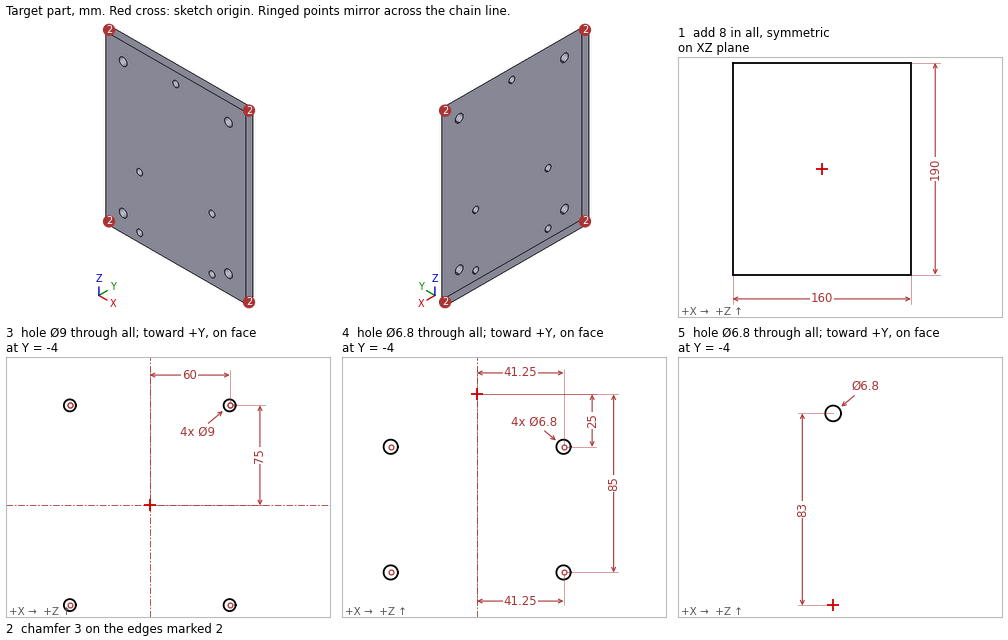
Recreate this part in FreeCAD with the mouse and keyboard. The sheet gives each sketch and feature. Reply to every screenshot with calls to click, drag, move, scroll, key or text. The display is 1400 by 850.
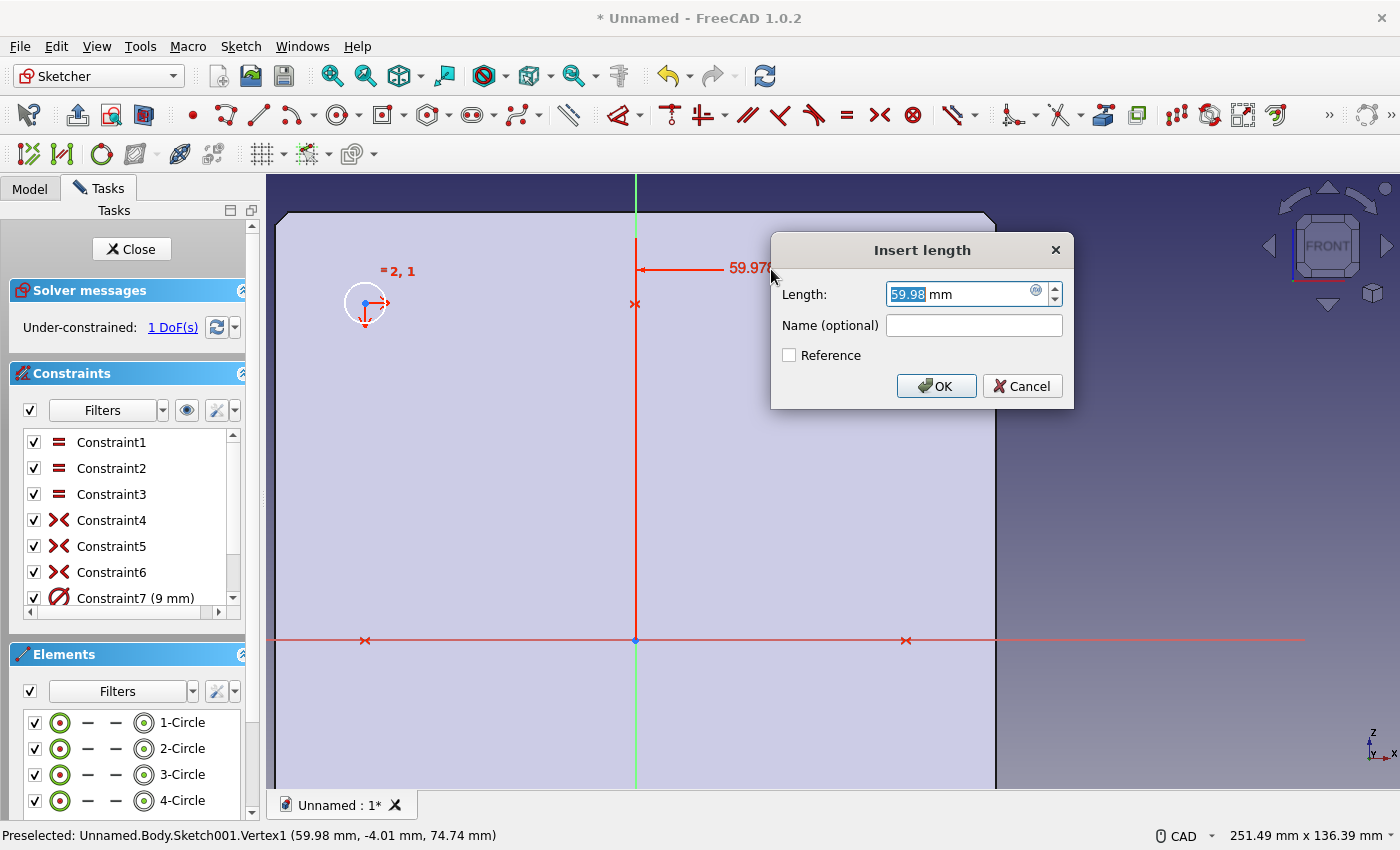
text(60)
key(Return)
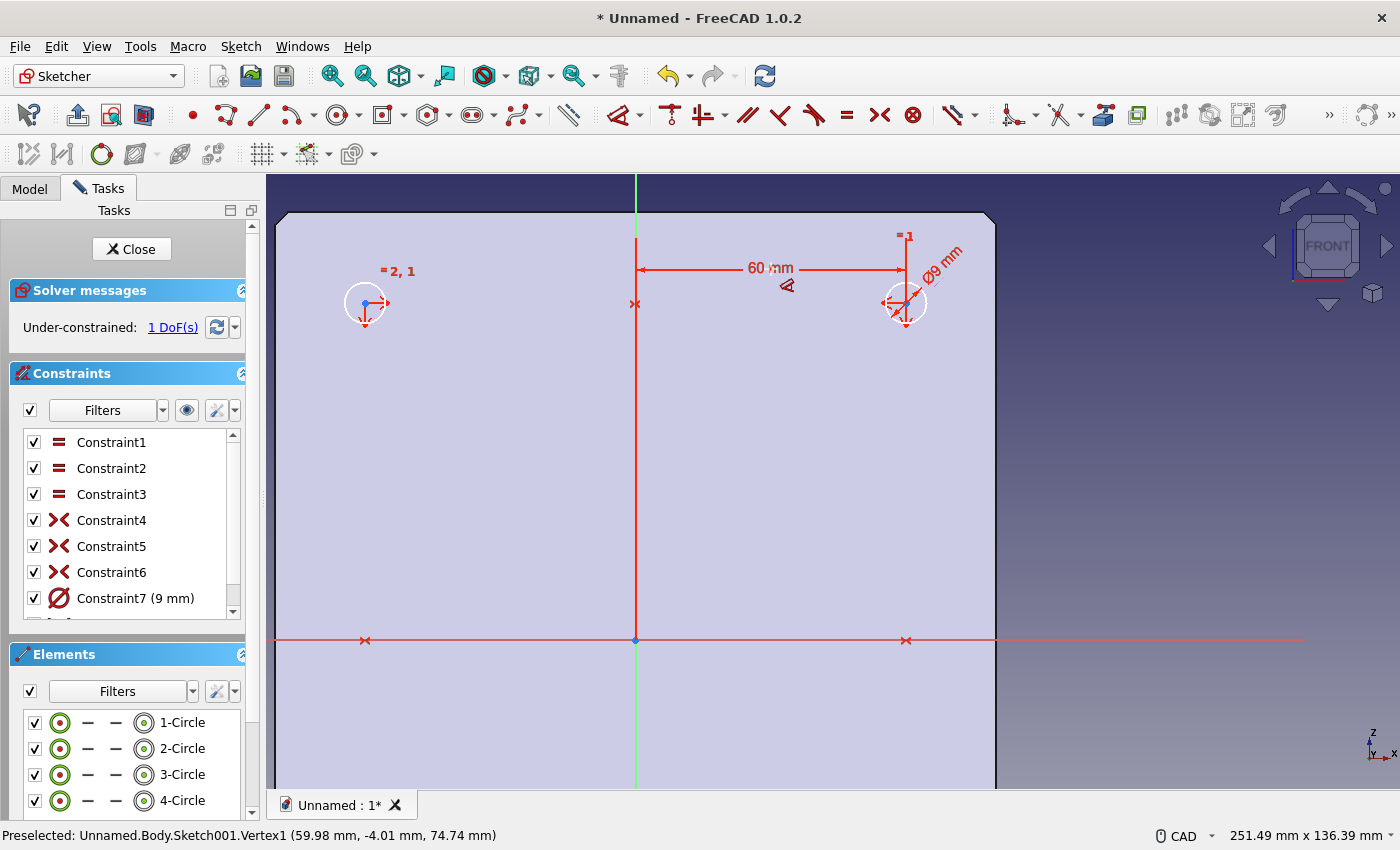
click(906, 303)
click(940, 472)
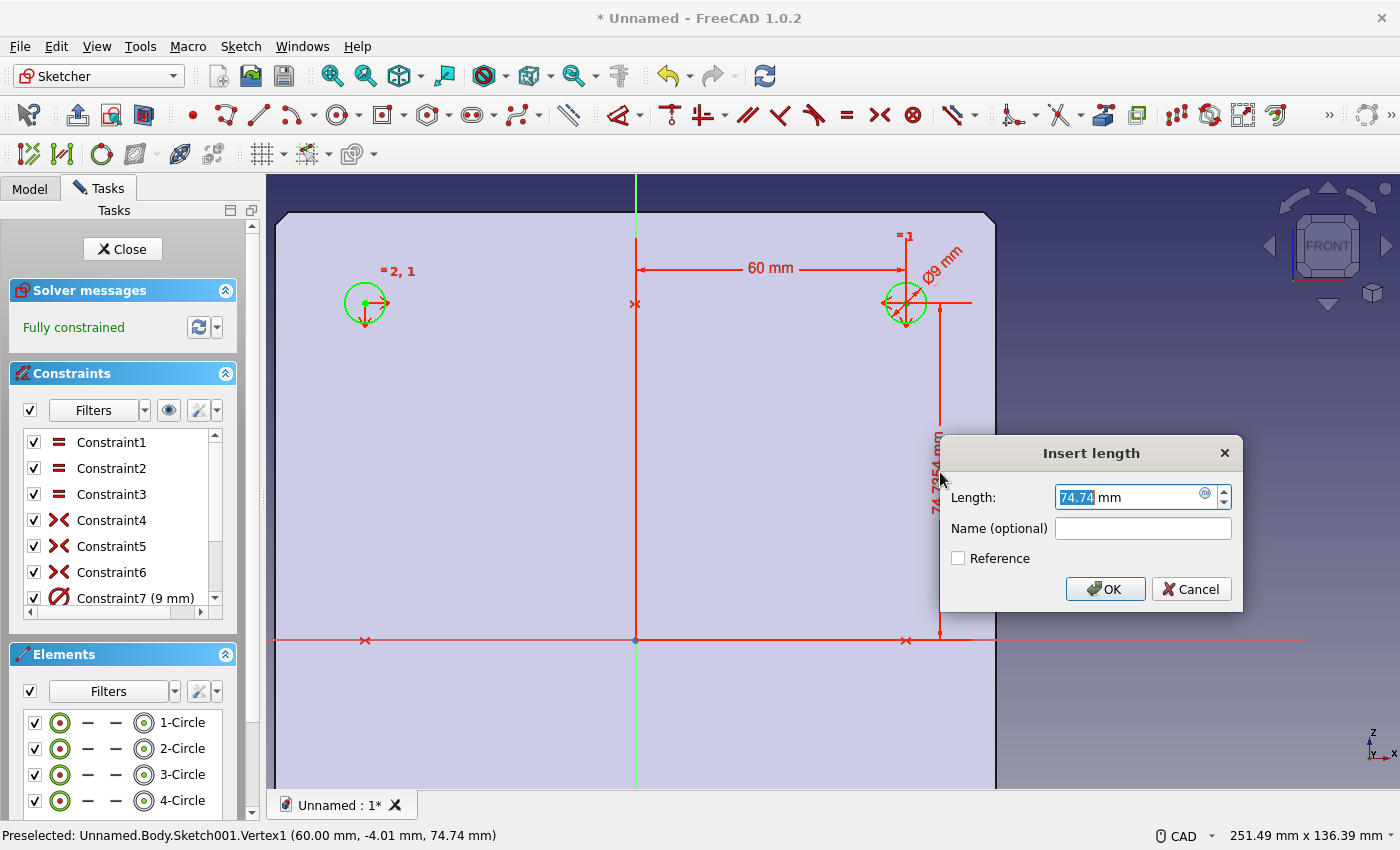
text(75)
key(Return)
key(Escape)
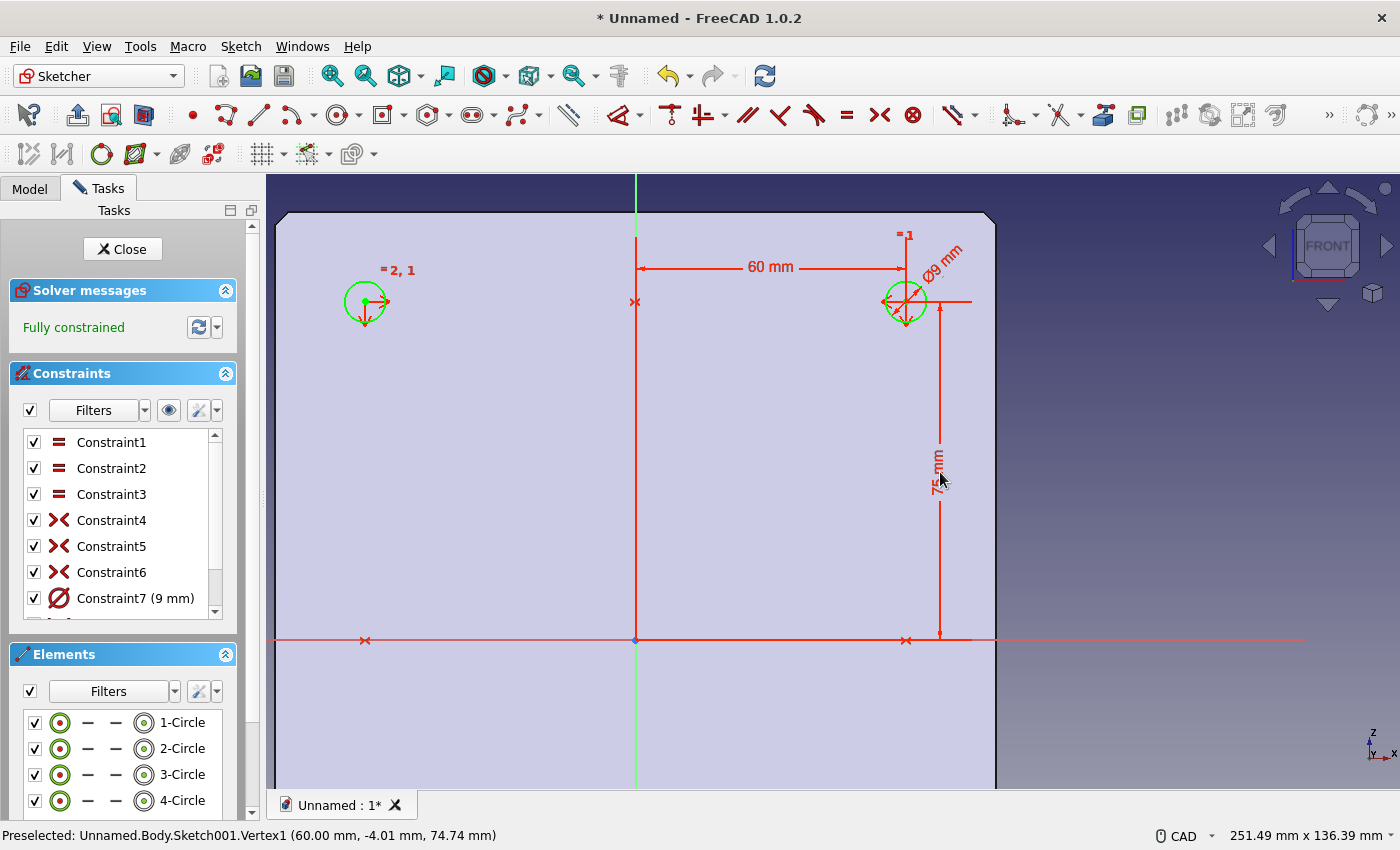
click(123, 249)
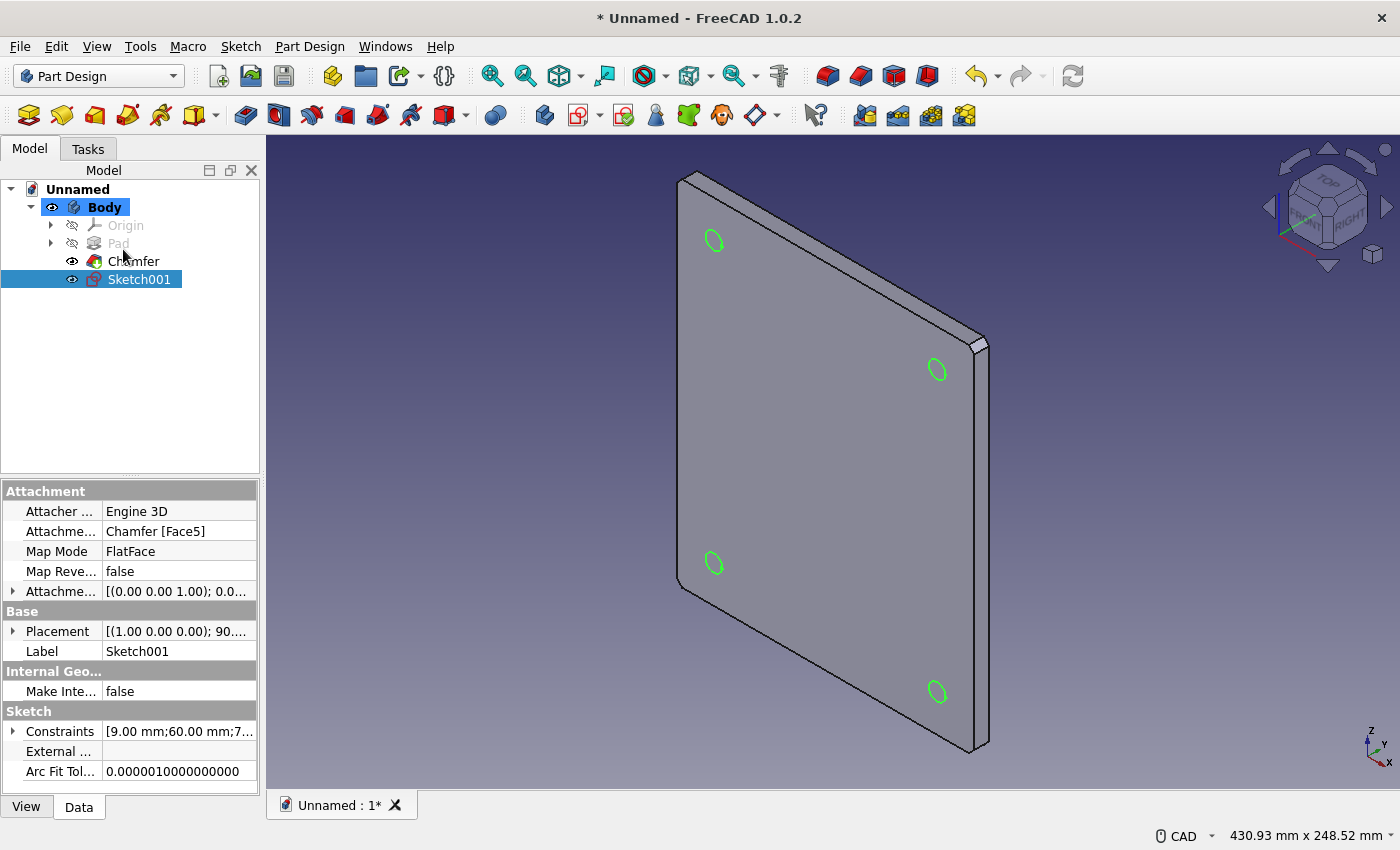
click(279, 116)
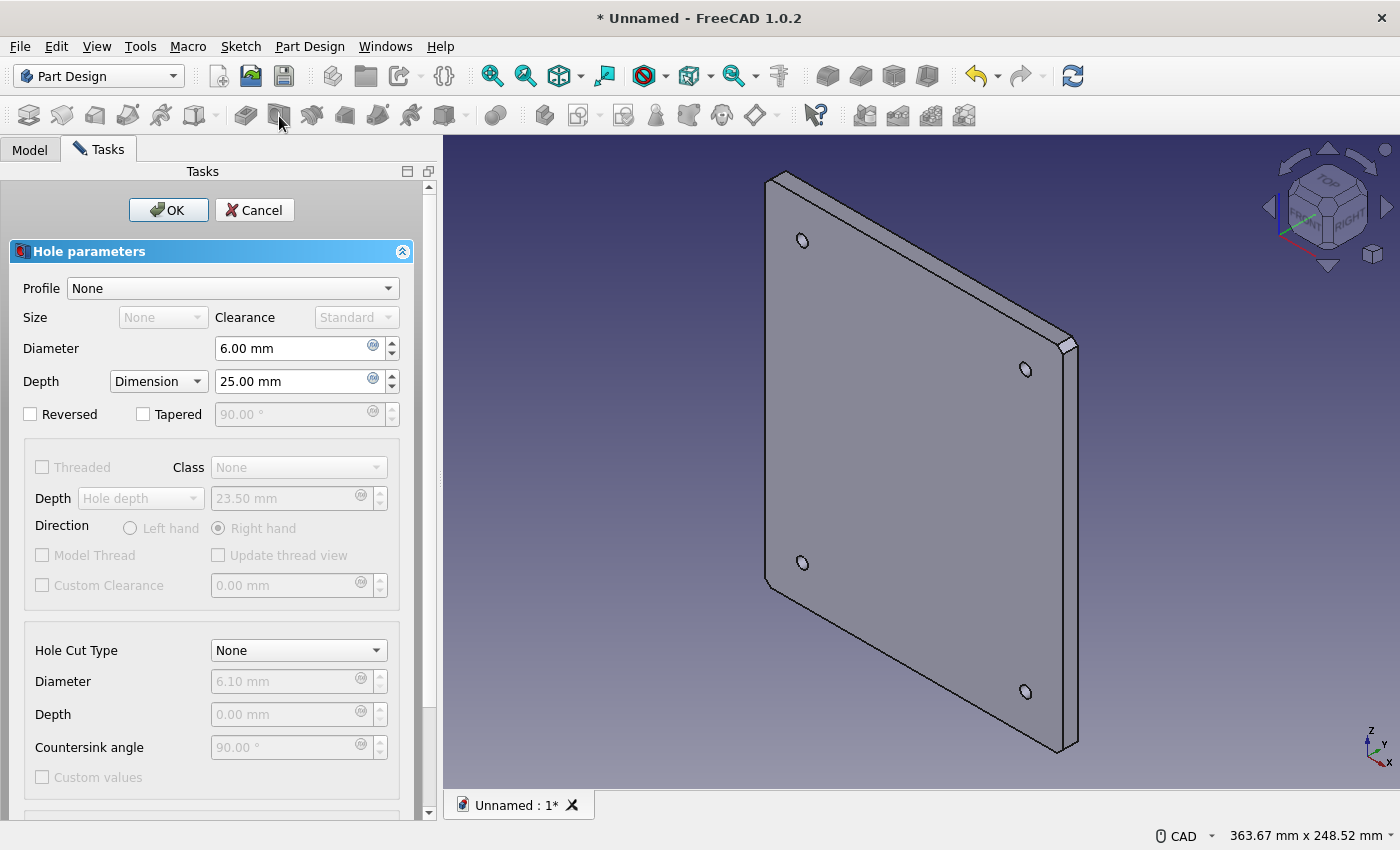
triple_click(300, 348)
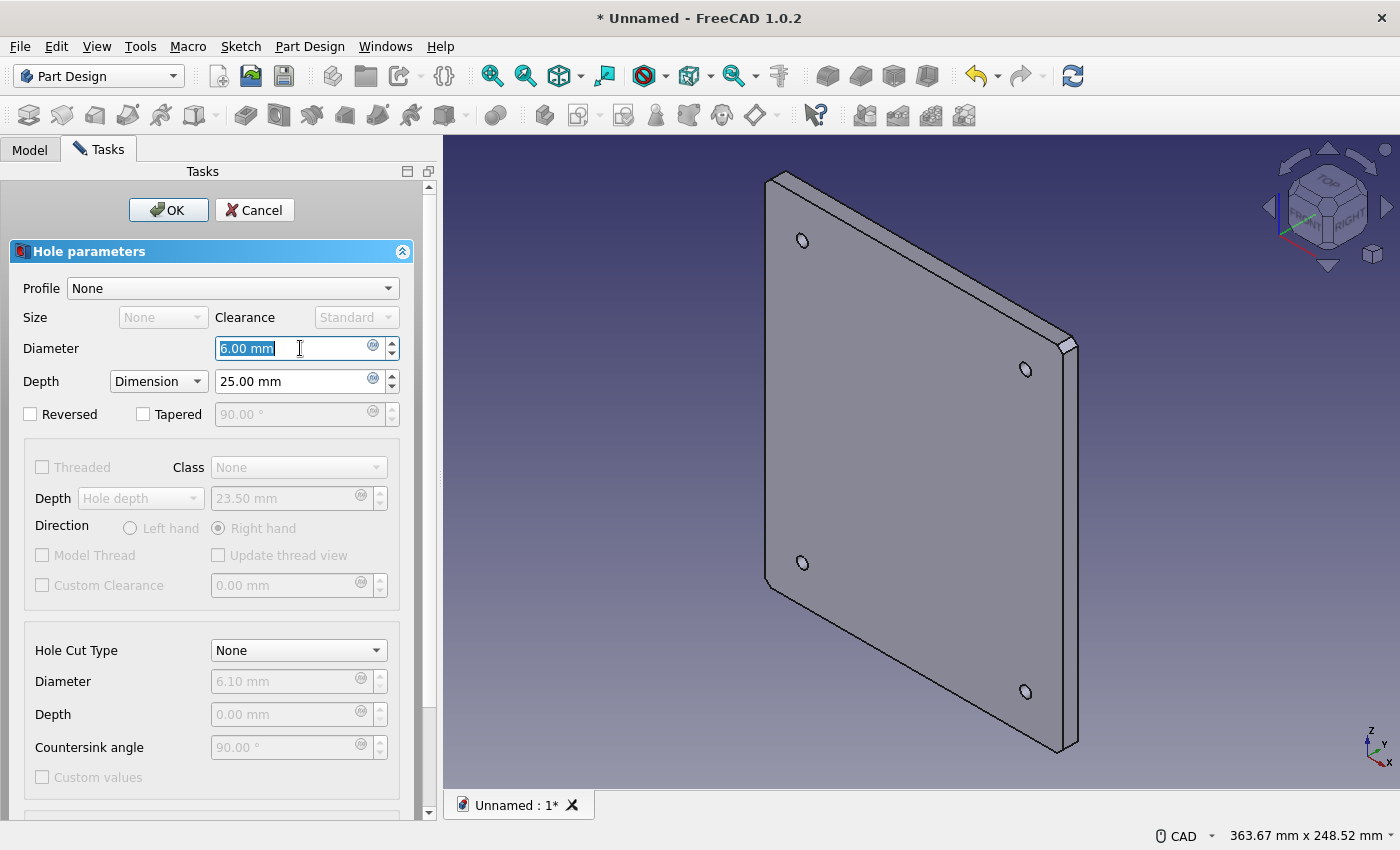
text(9)
key(Tab)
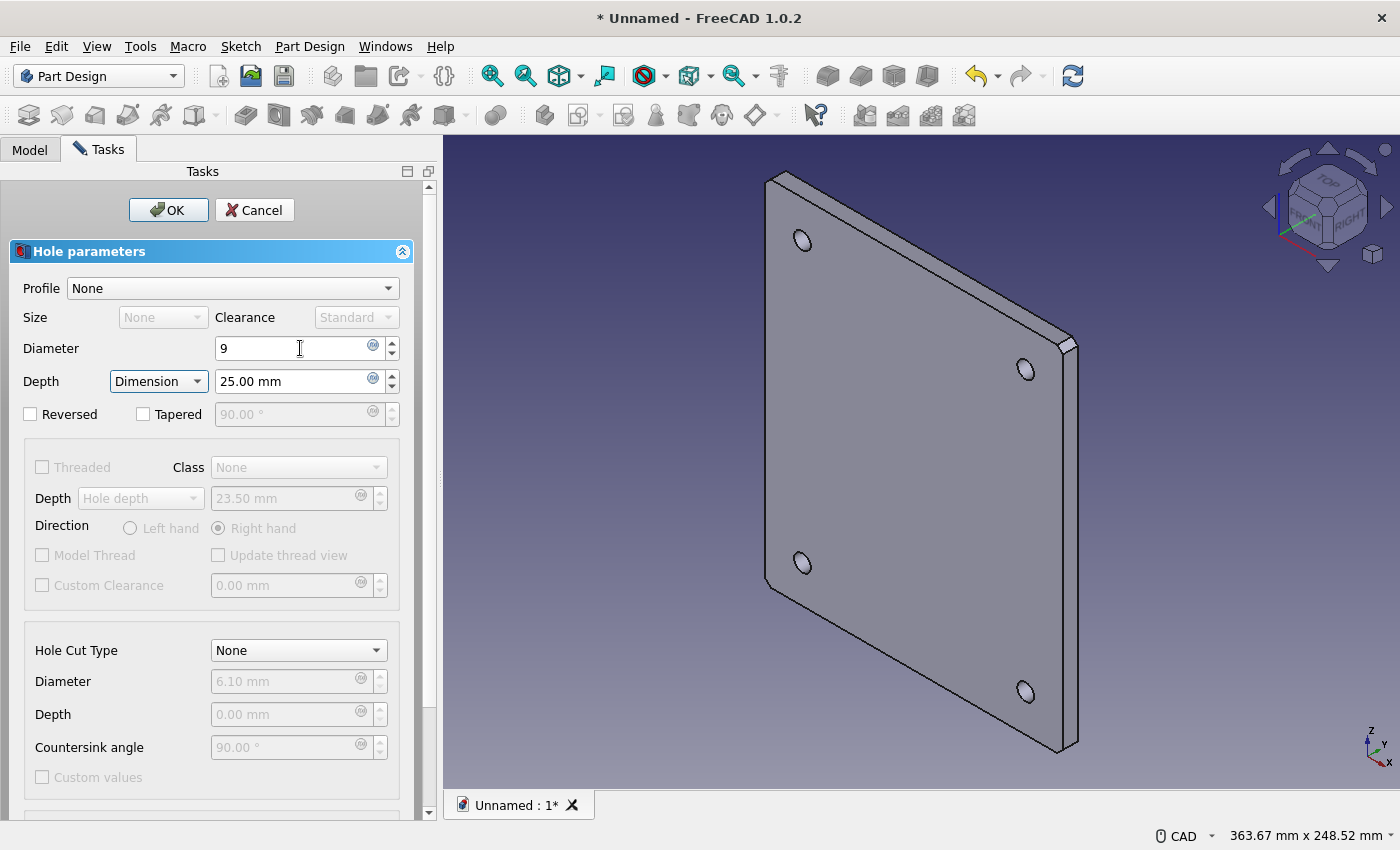
click(160, 382)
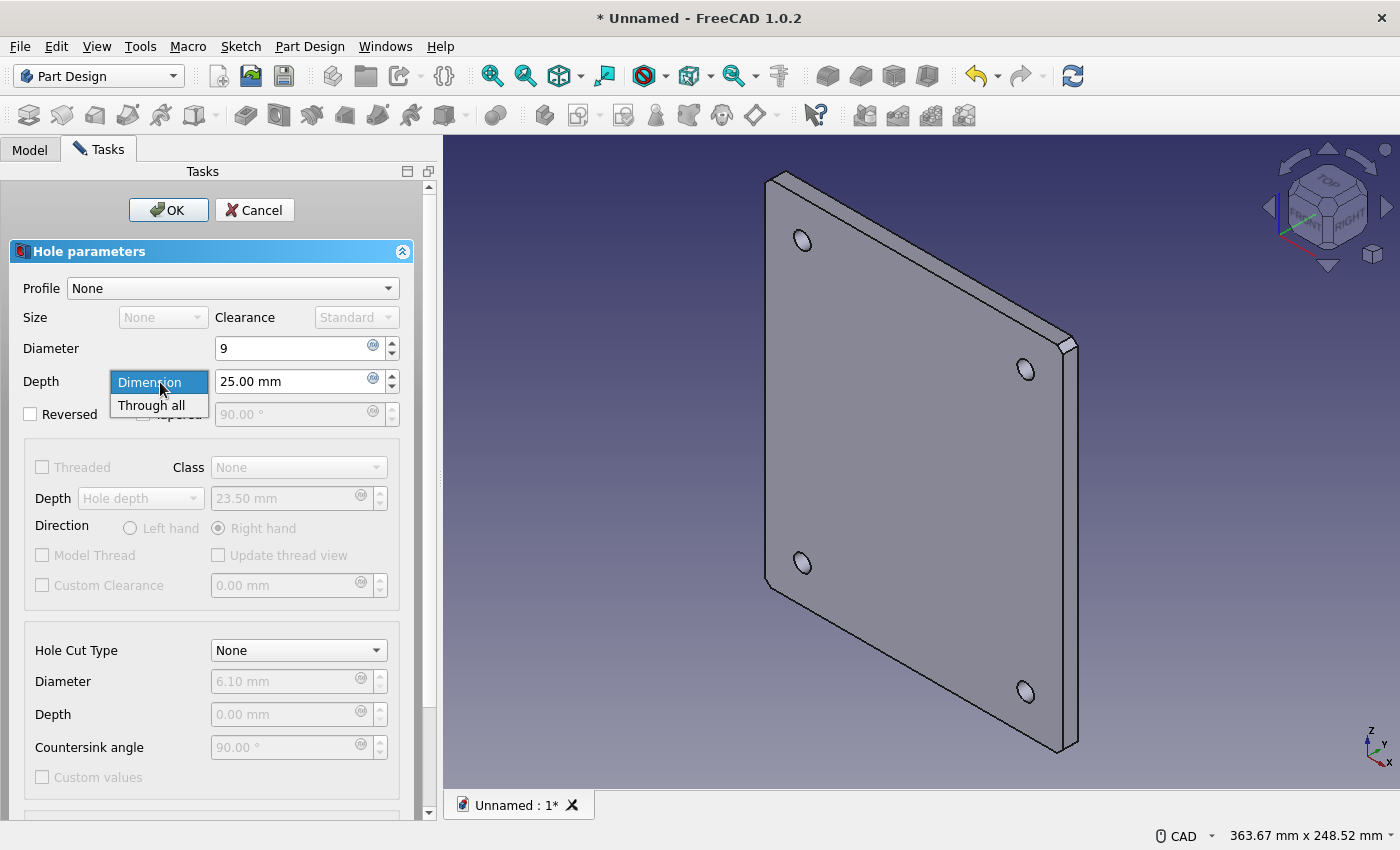
click(158, 406)